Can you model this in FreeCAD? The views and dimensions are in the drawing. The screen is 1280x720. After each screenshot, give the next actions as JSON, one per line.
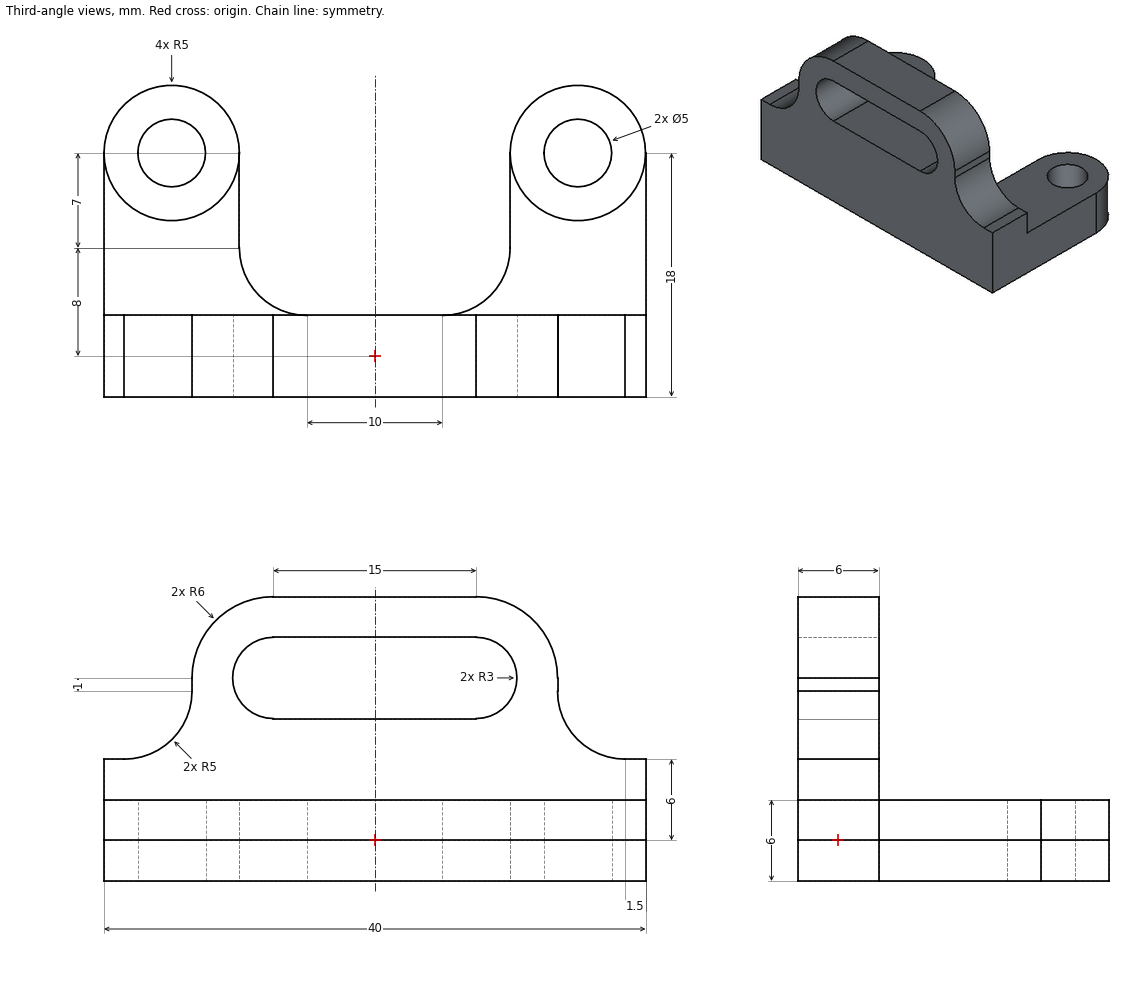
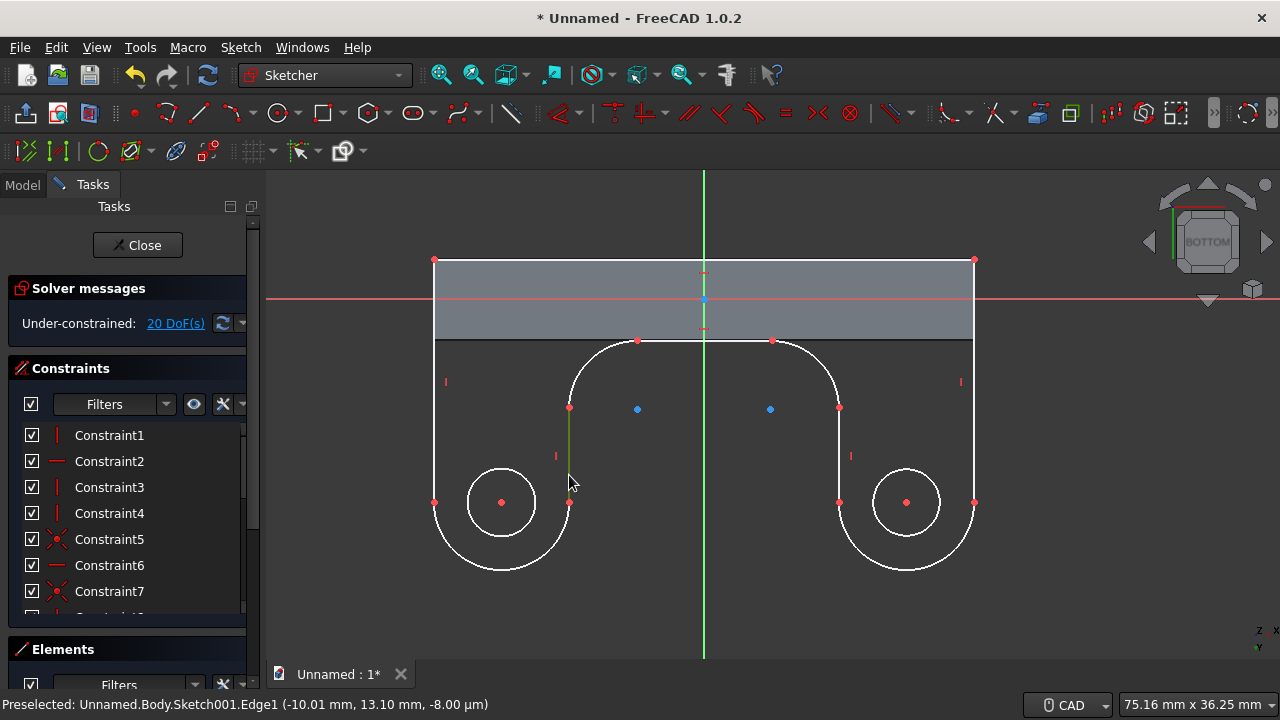
{"action": "left_click", "coordinate": [606, 348]}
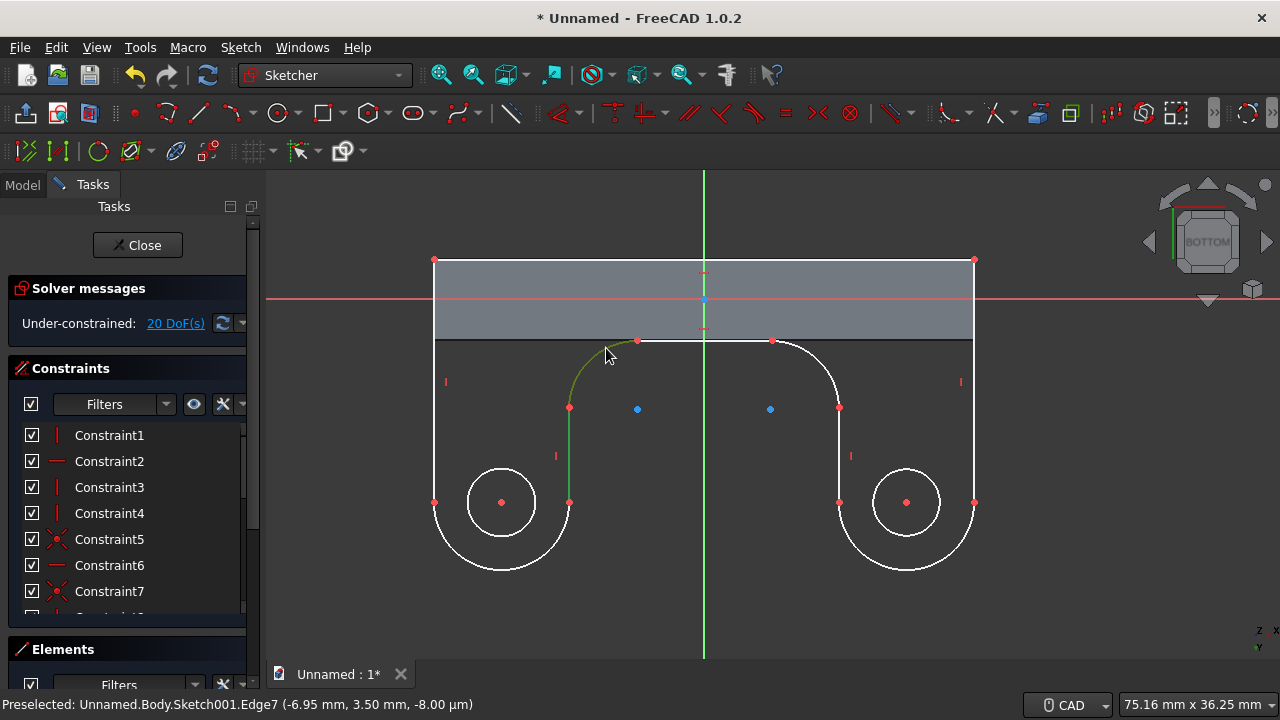
{"action": "left_click", "coordinate": [754, 114]}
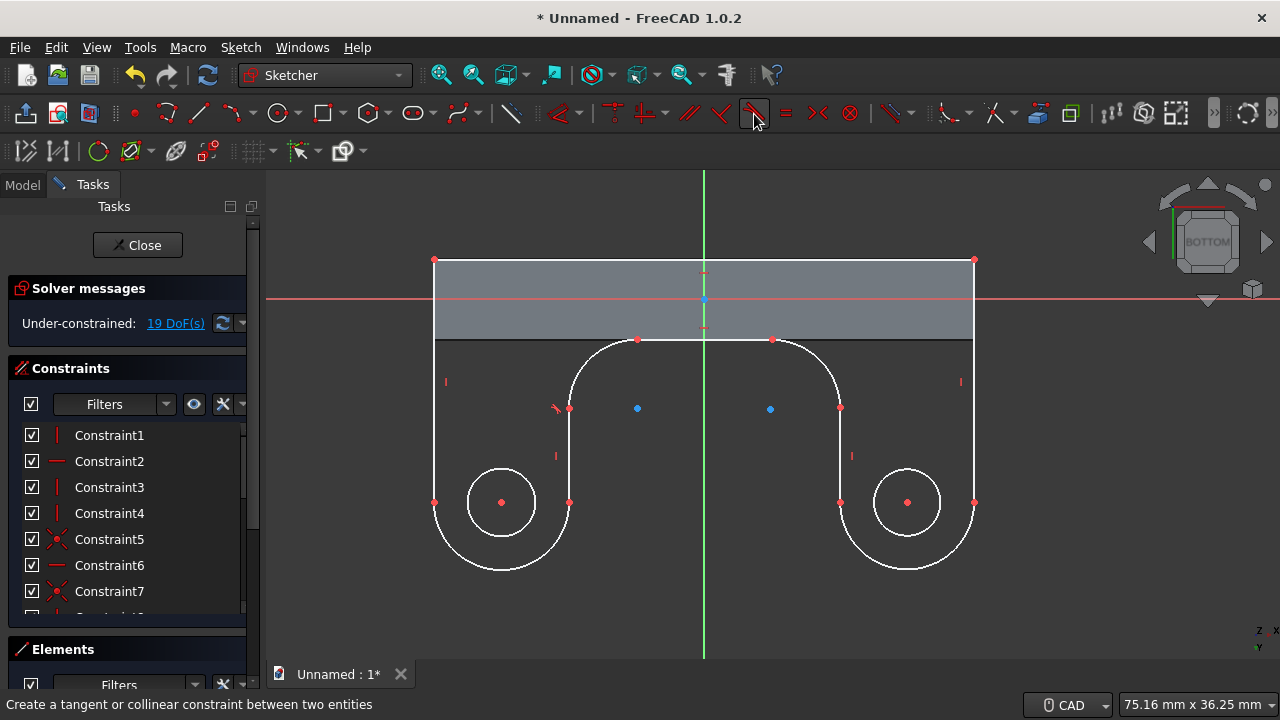
{"action": "left_click", "coordinate": [569, 475]}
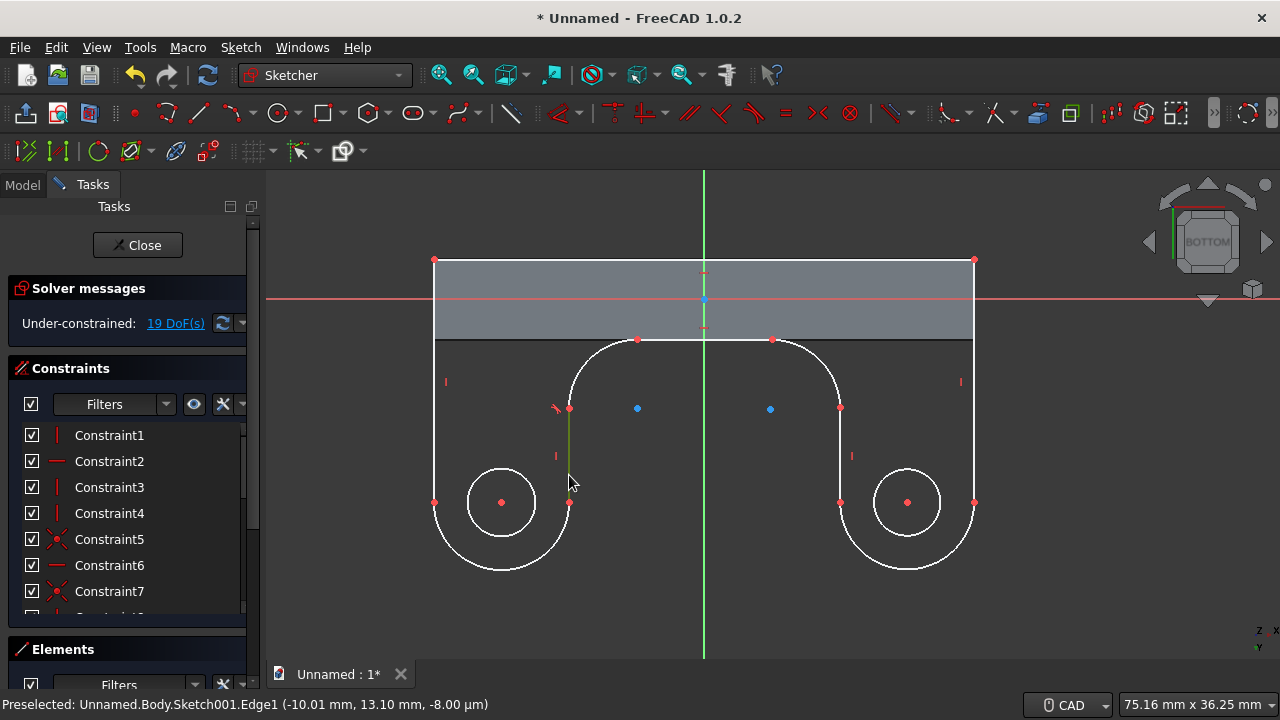
{"action": "left_click", "coordinate": [462, 557]}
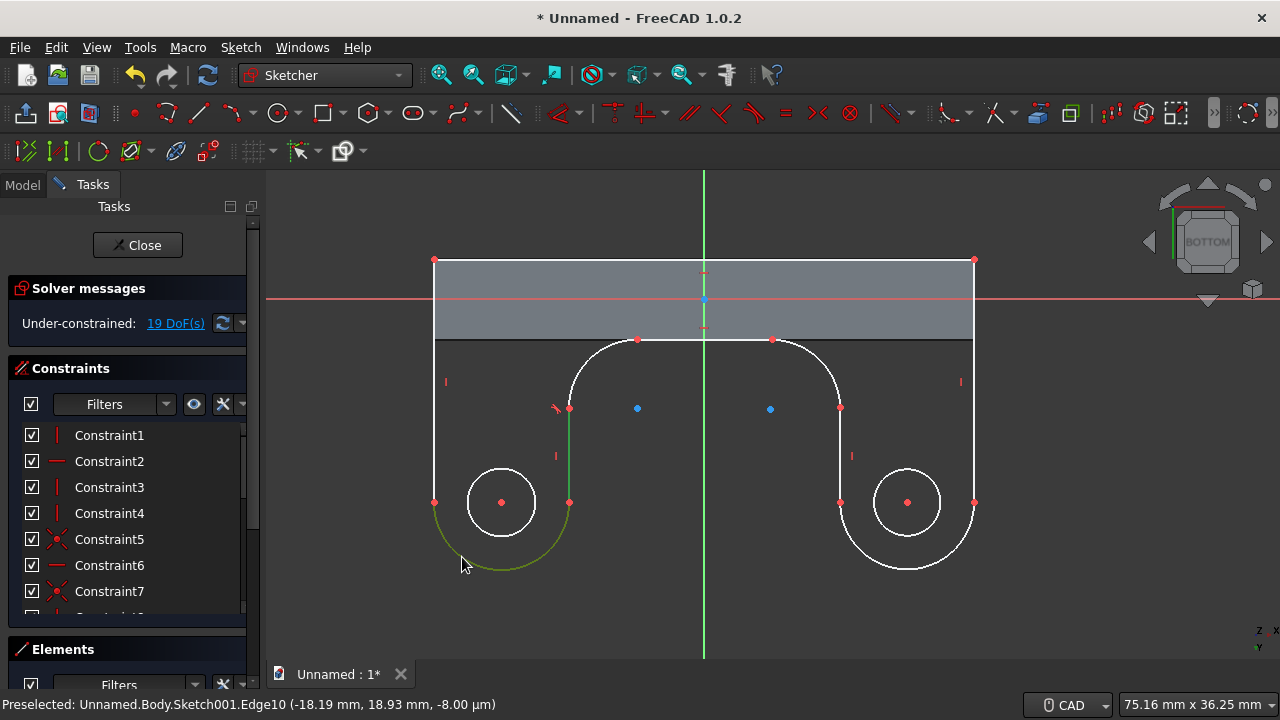
{"action": "left_click", "coordinate": [754, 114]}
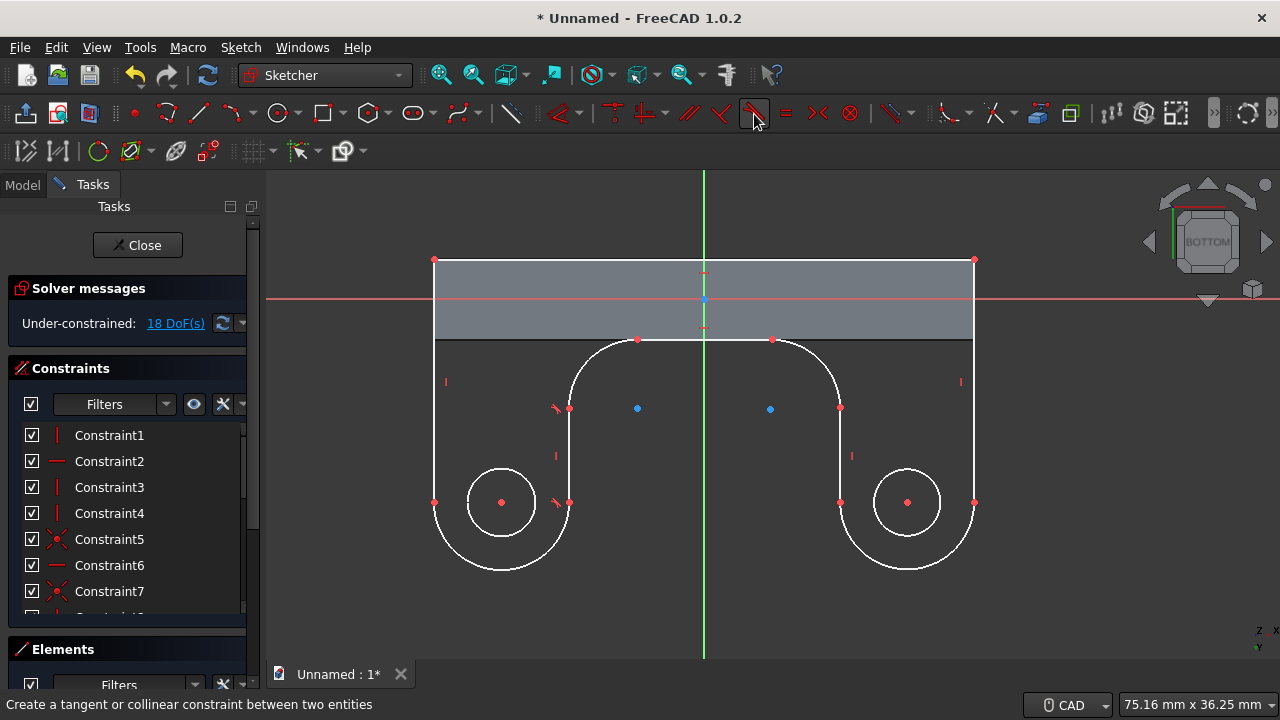
{"action": "left_click", "coordinate": [678, 340]}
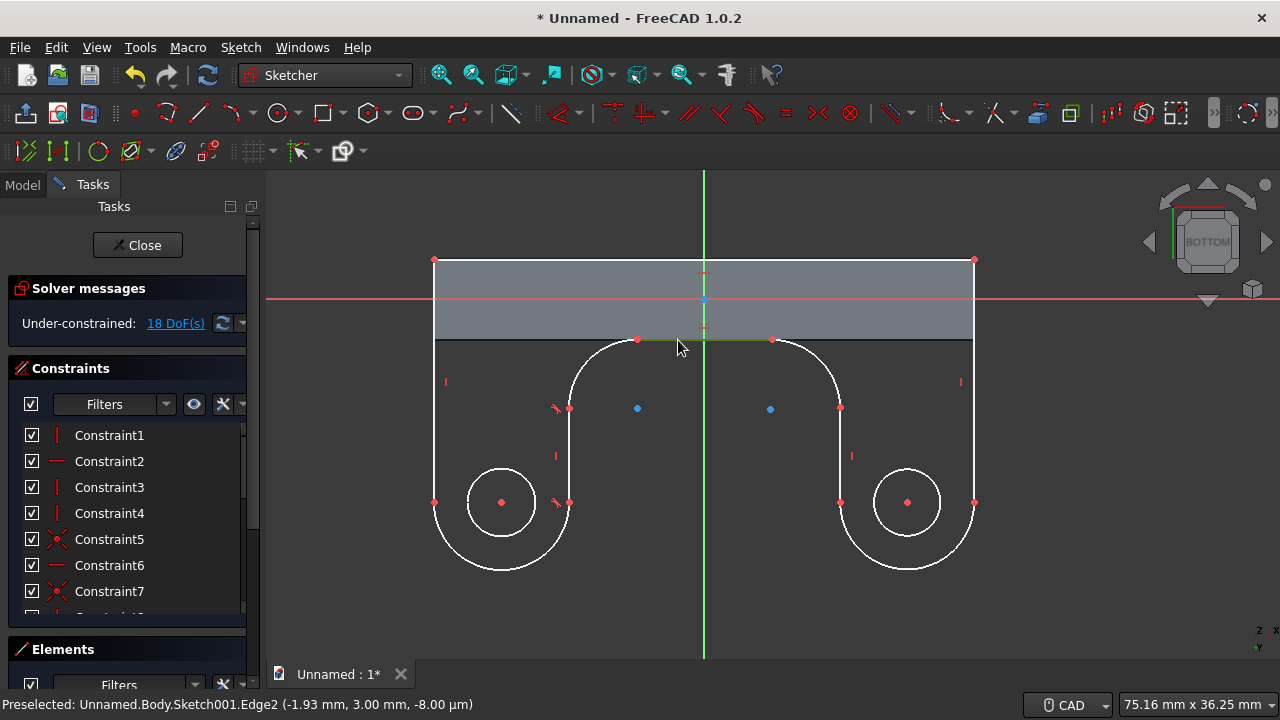
{"action": "left_click", "coordinate": [606, 347]}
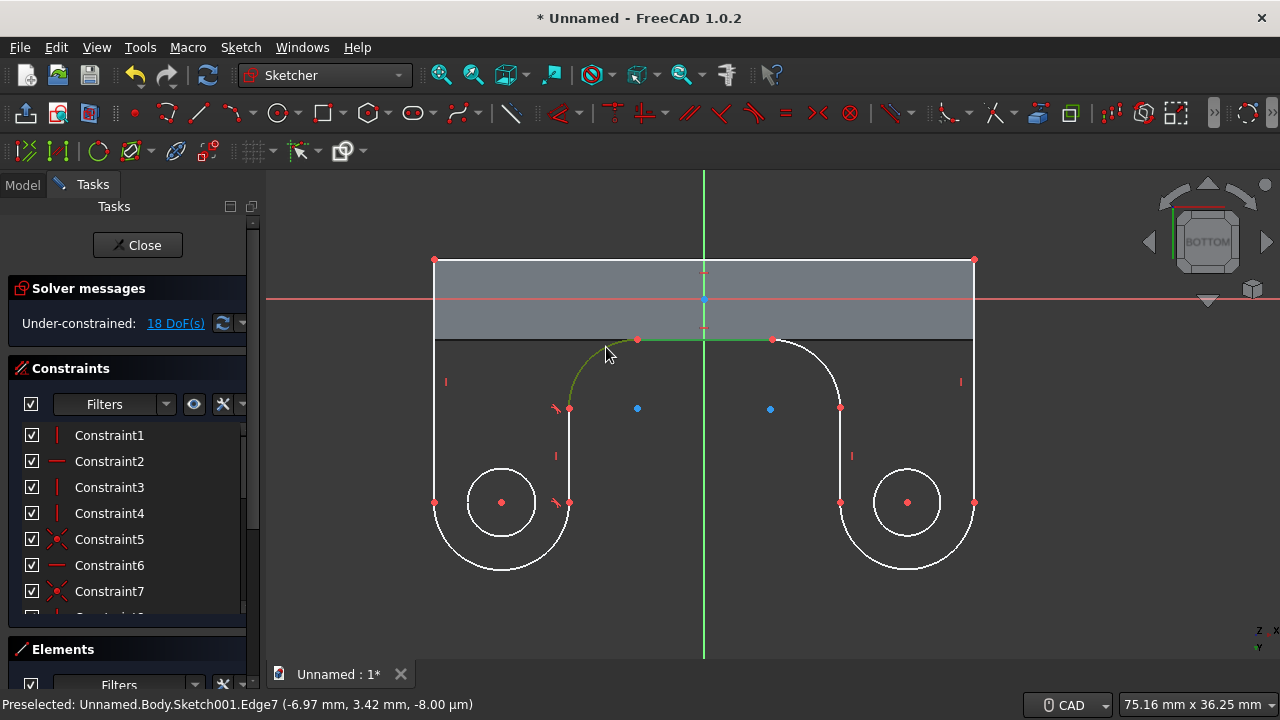
{"action": "left_click", "coordinate": [754, 114]}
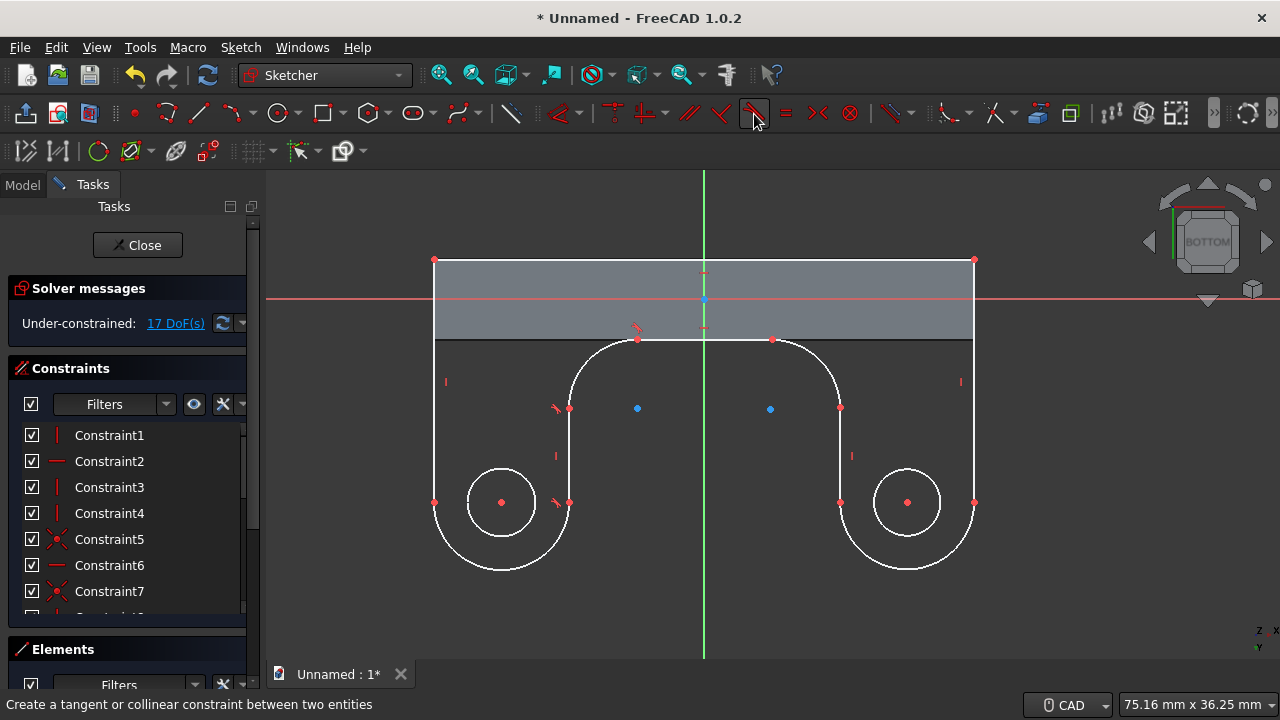
{"action": "left_click", "coordinate": [678, 340]}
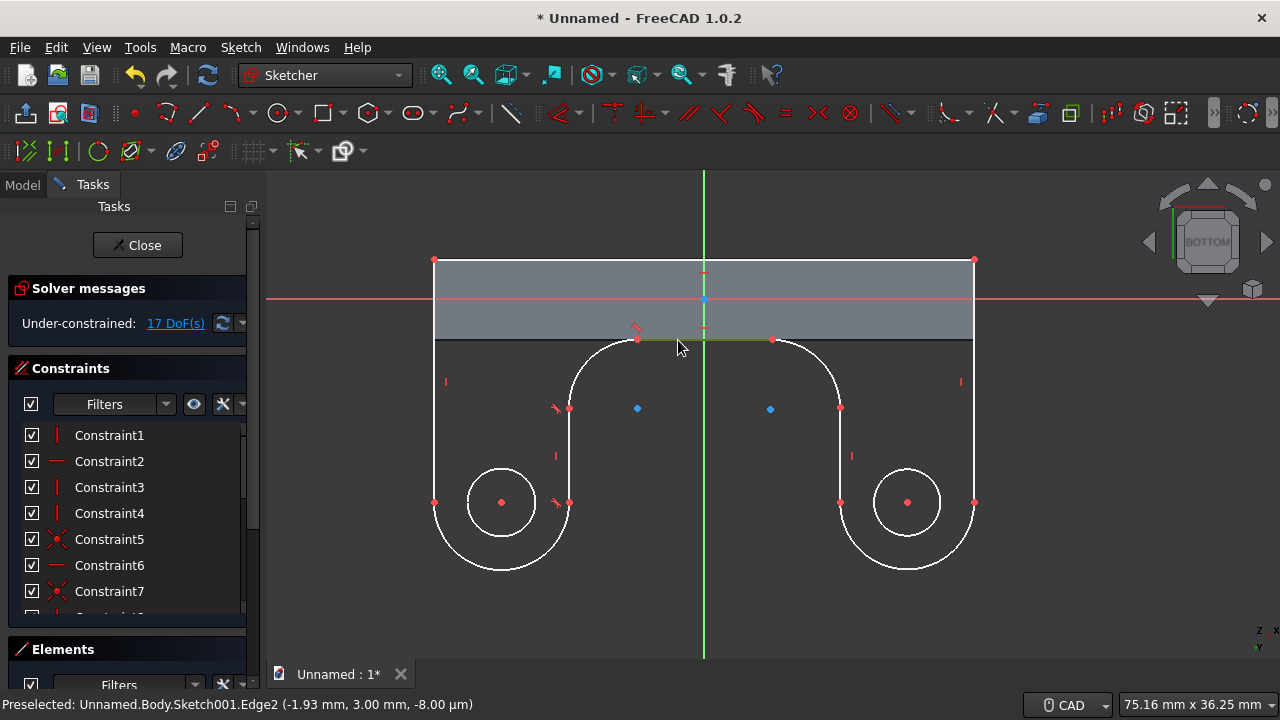
{"action": "left_click", "coordinate": [832, 377]}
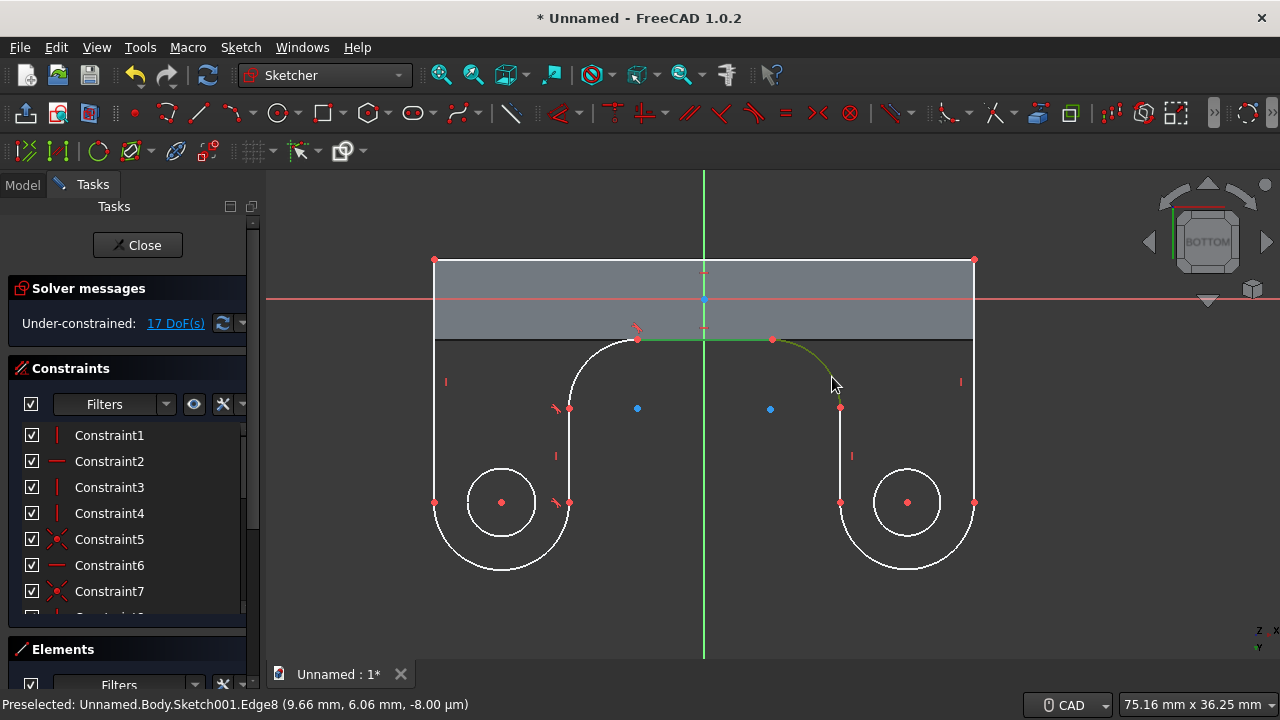
{"action": "left_click", "coordinate": [754, 114]}